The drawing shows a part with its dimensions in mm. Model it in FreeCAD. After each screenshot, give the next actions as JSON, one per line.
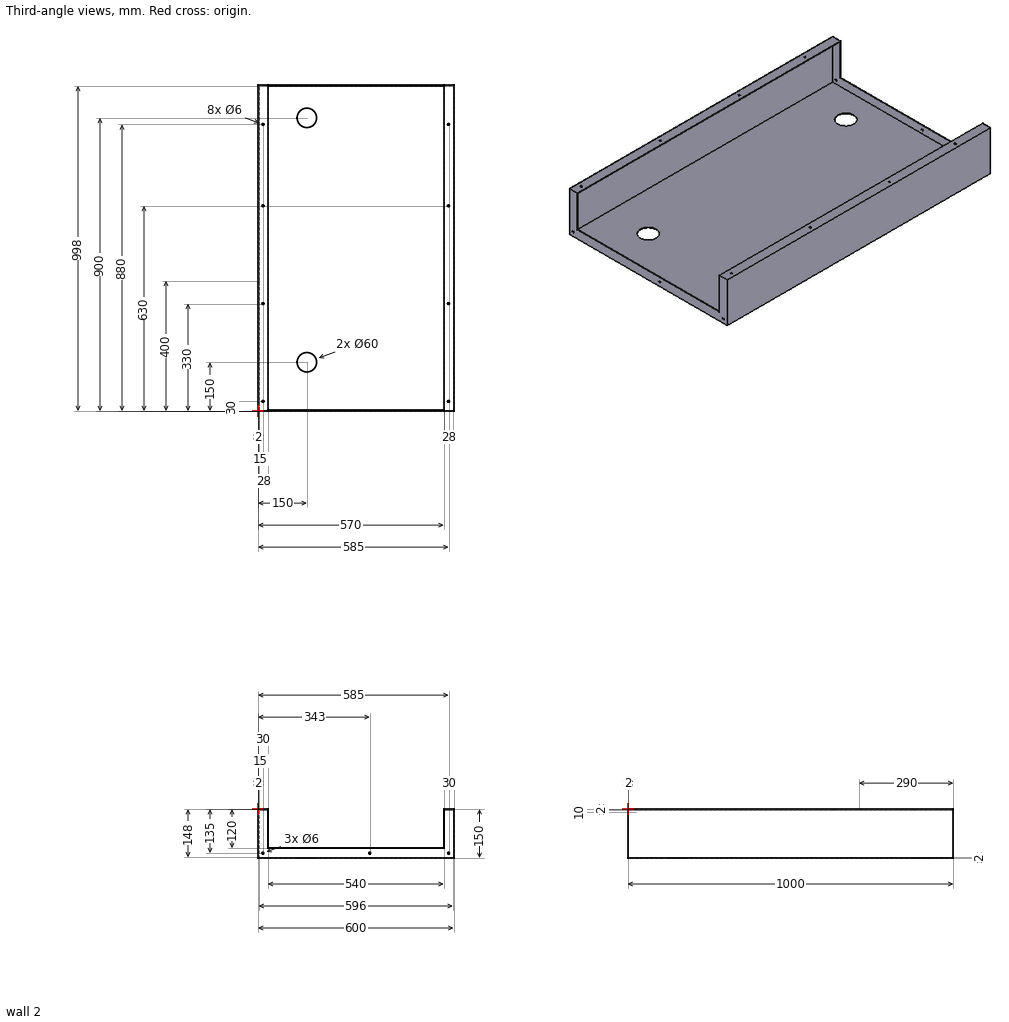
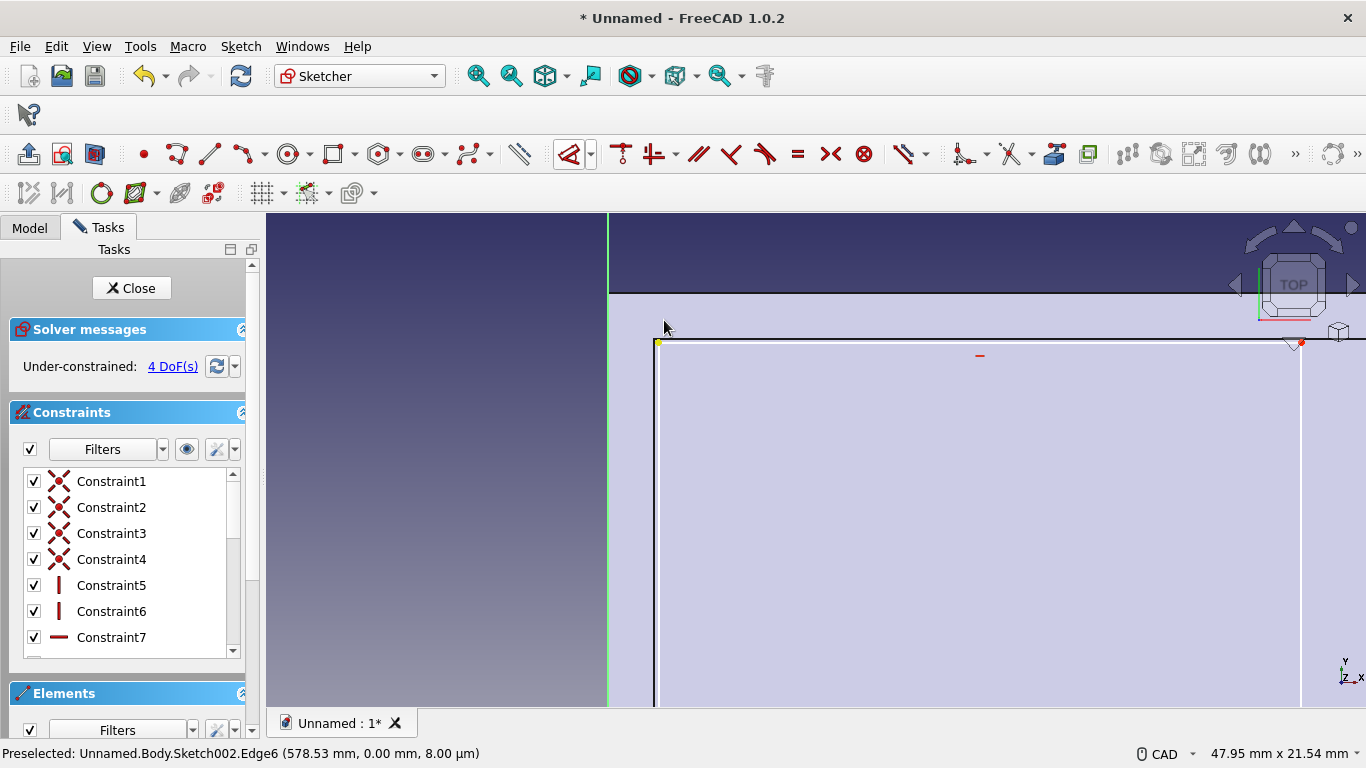
{"action": "left_click", "coordinate": [659, 343]}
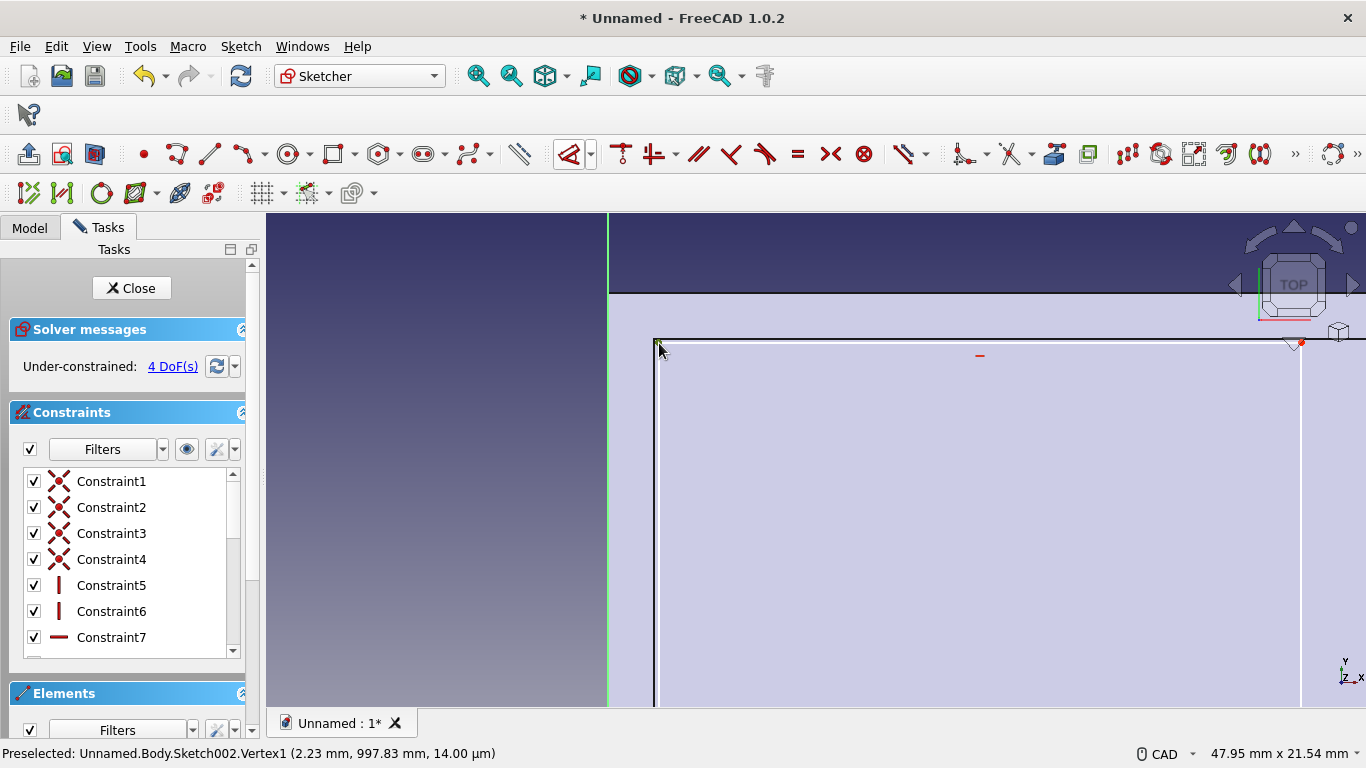
{"action": "left_click", "coordinate": [590, 154]}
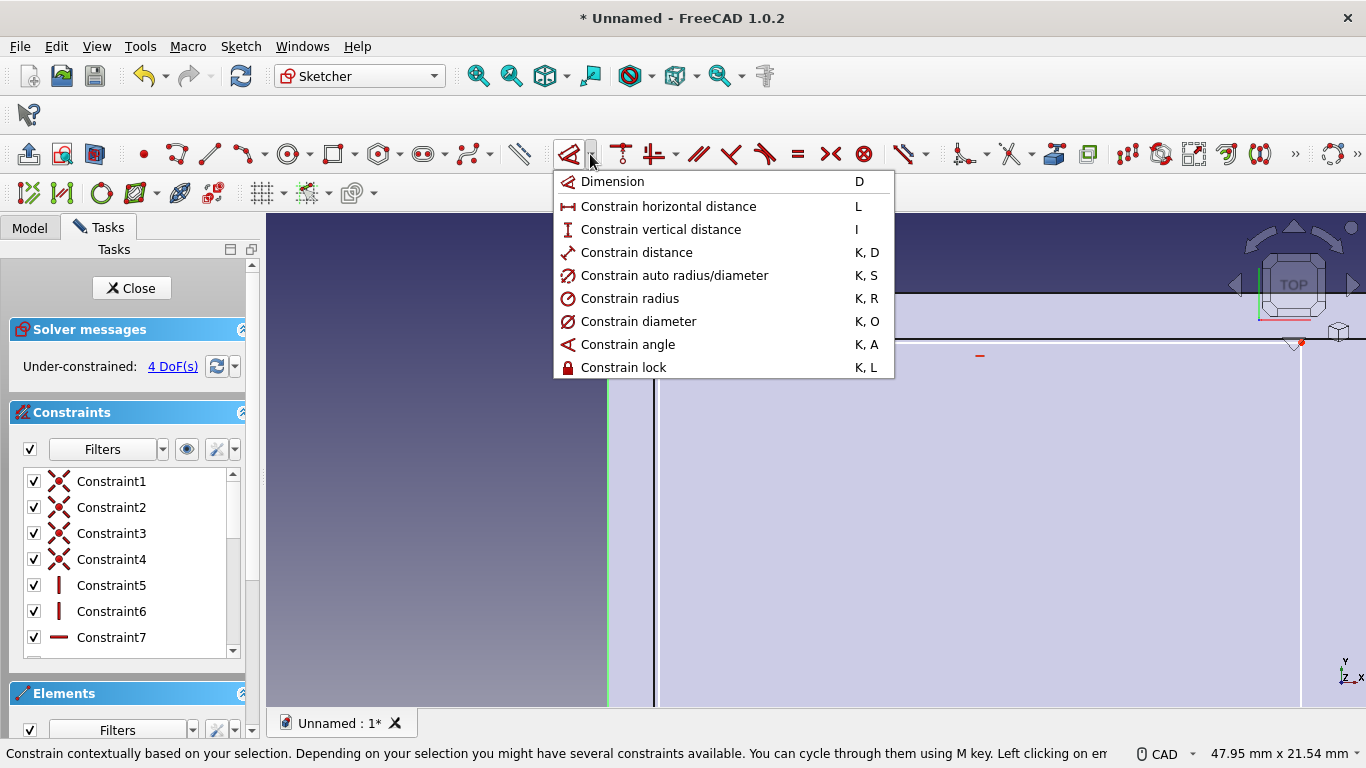
{"action": "left_click", "coordinate": [724, 206]}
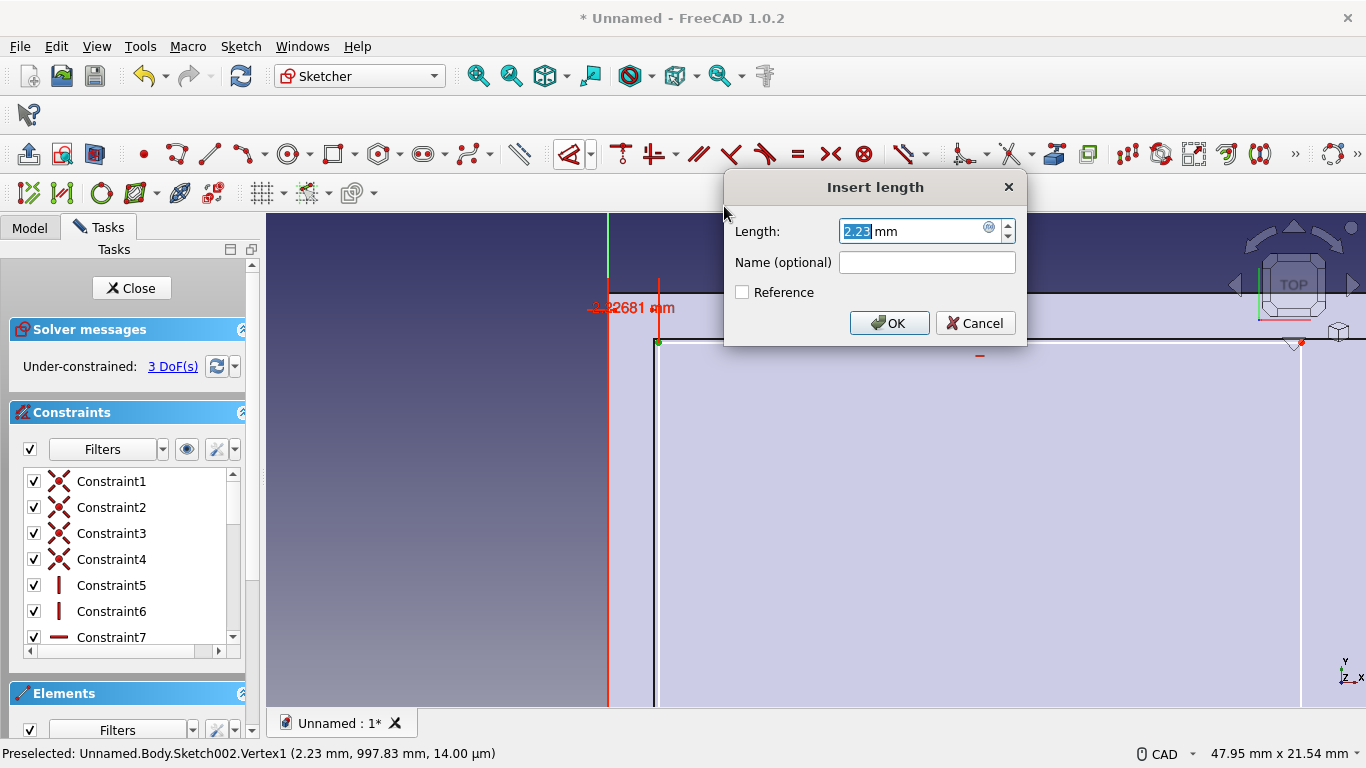
{"action": "type", "text": "2"}
{"action": "key", "text": "Return"}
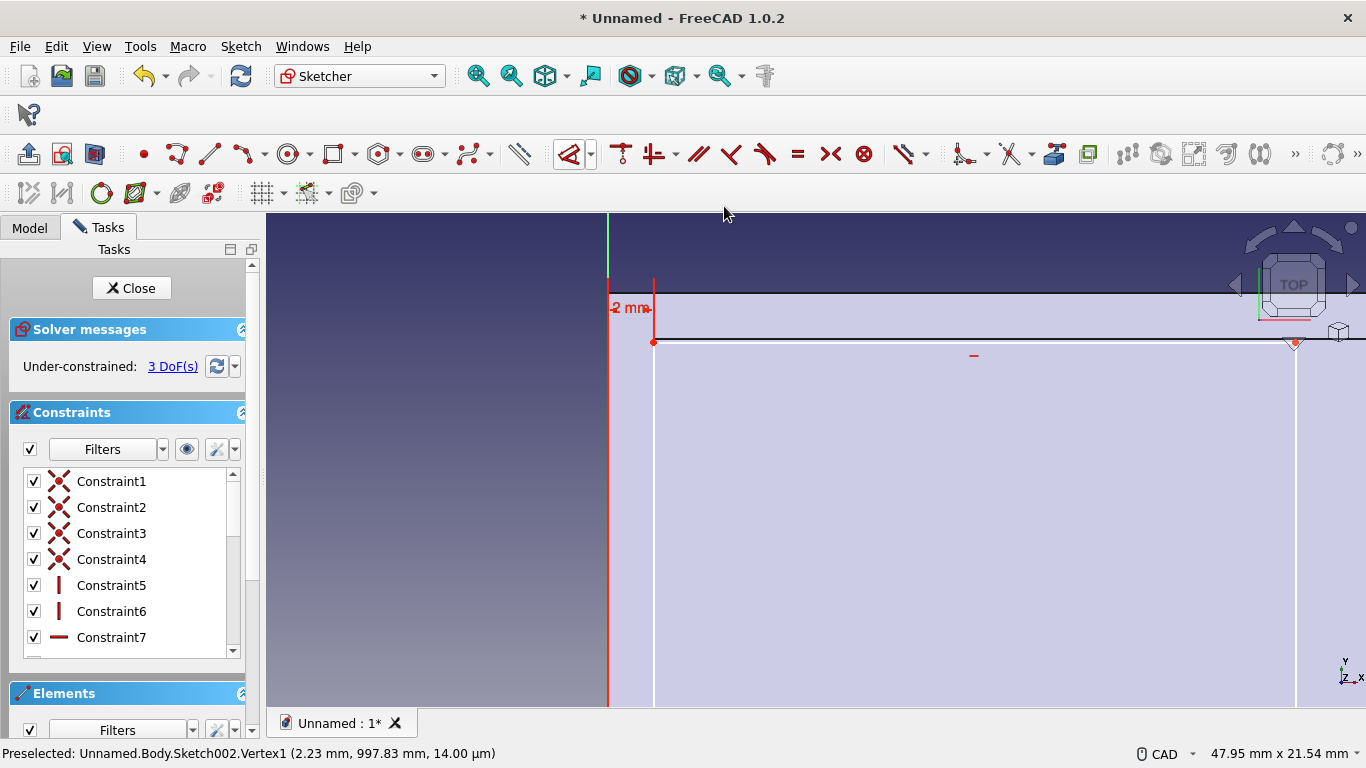
{"action": "scroll", "coordinate": [748, 460], "scroll_direction": "down", "scroll_amount": 15}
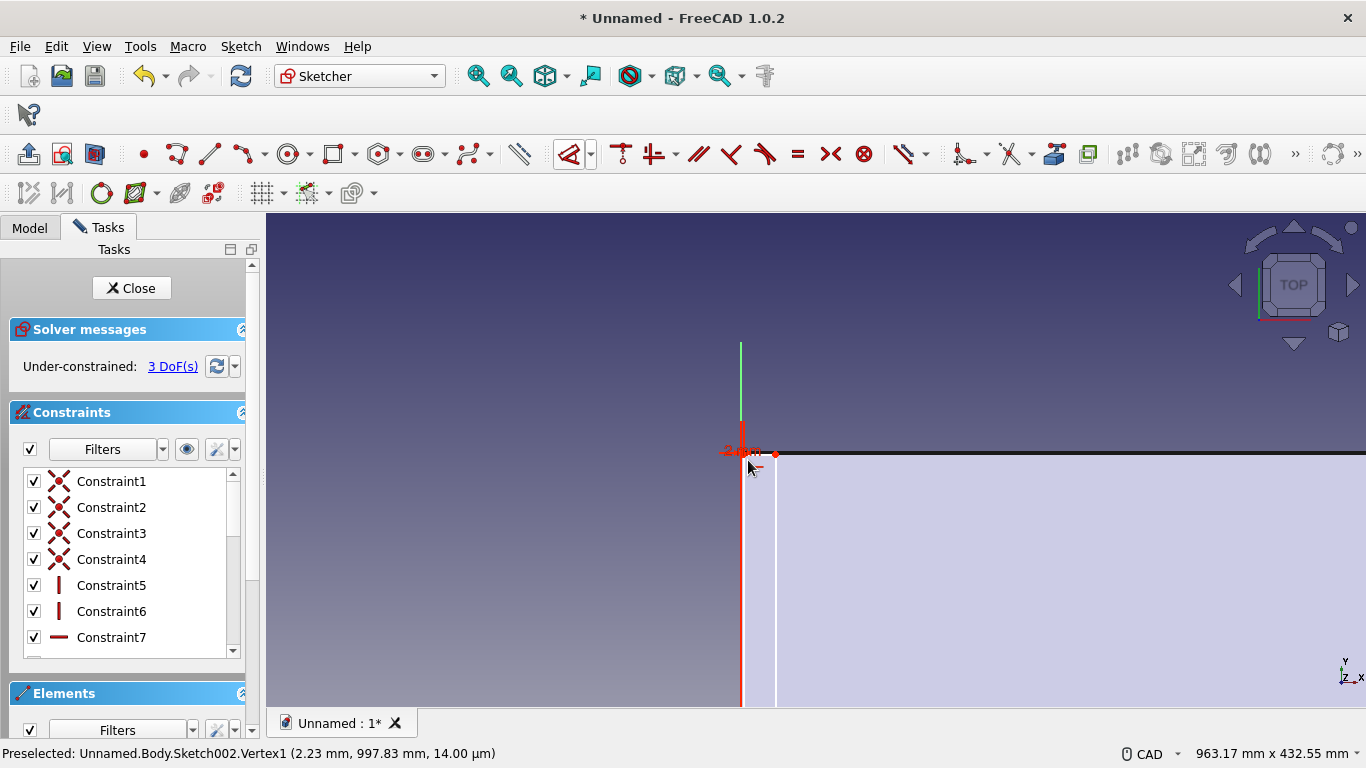
{"action": "scroll", "coordinate": [638, 275], "scroll_direction": "down", "scroll_amount": 7}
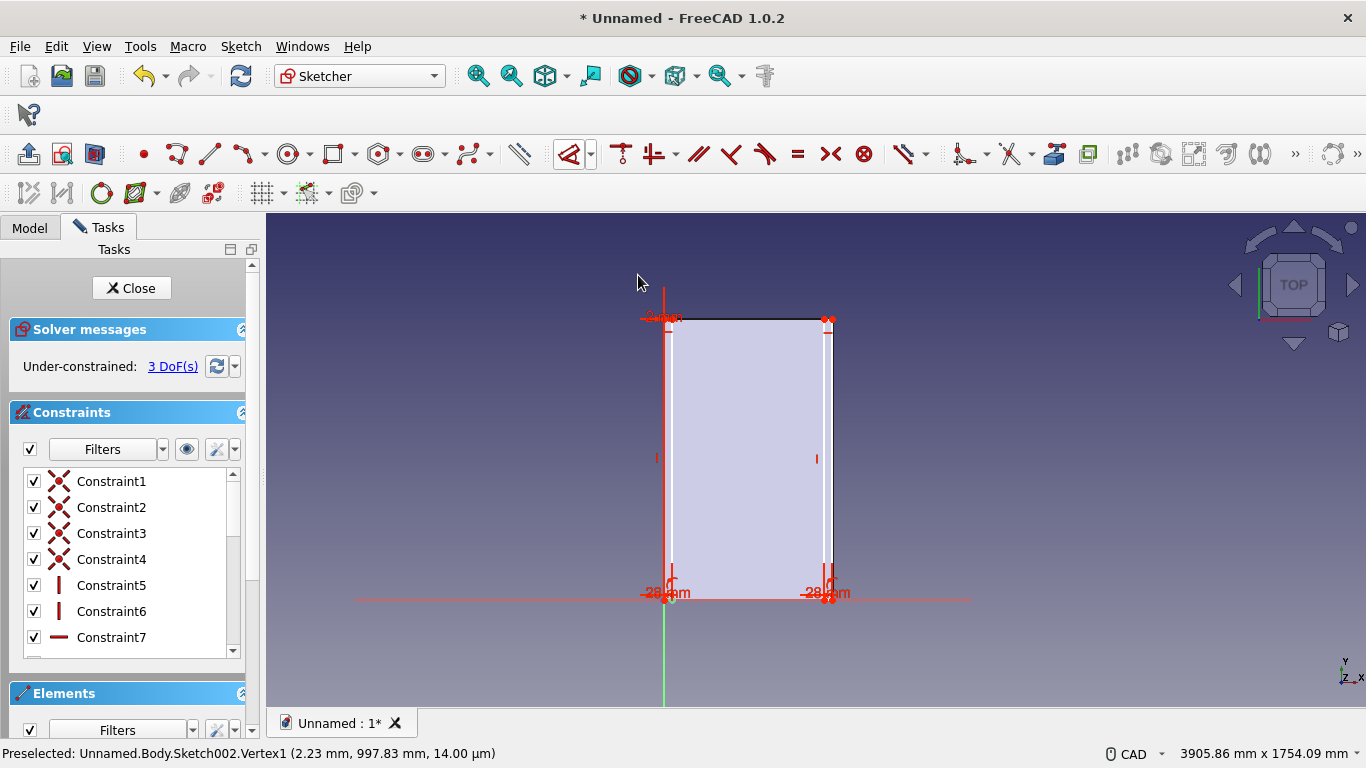
{"action": "scroll", "coordinate": [664, 404], "scroll_direction": "up", "scroll_amount": 14}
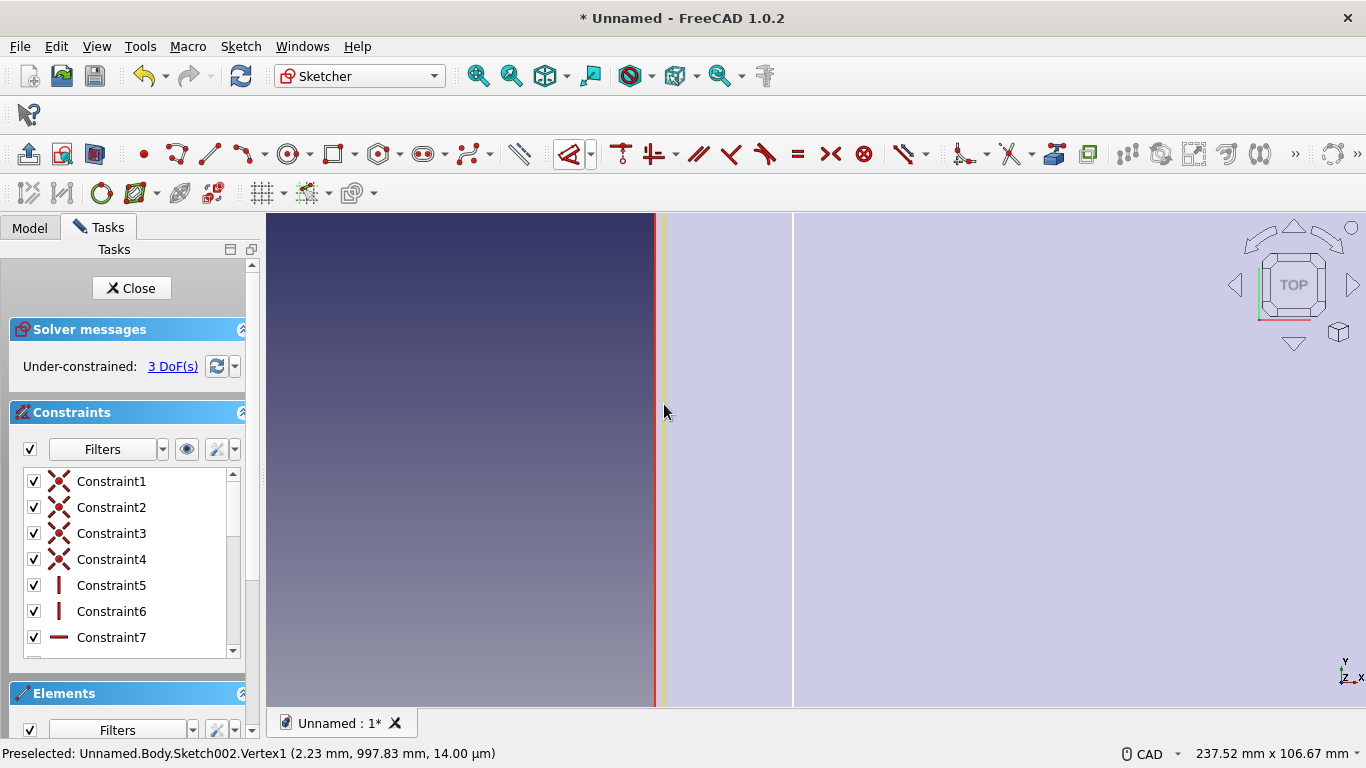
{"action": "left_click", "coordinate": [664, 393]}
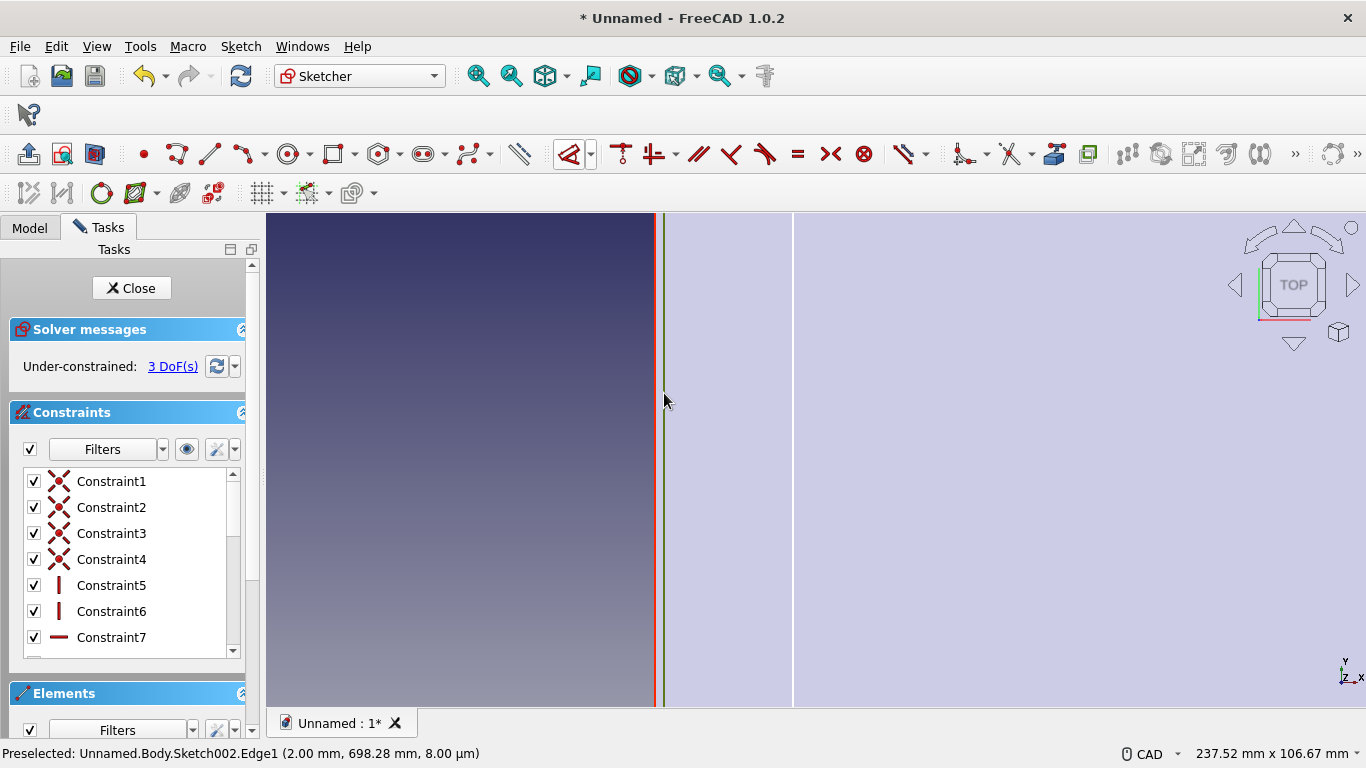
{"action": "left_click", "coordinate": [590, 154]}